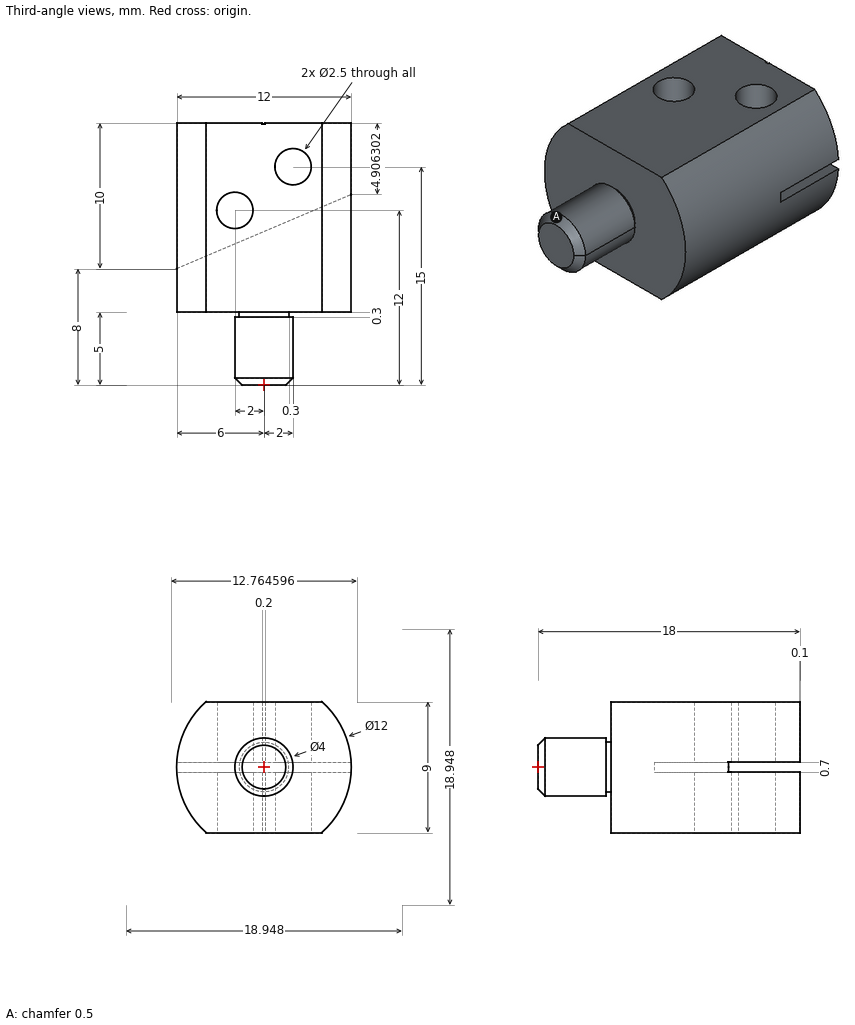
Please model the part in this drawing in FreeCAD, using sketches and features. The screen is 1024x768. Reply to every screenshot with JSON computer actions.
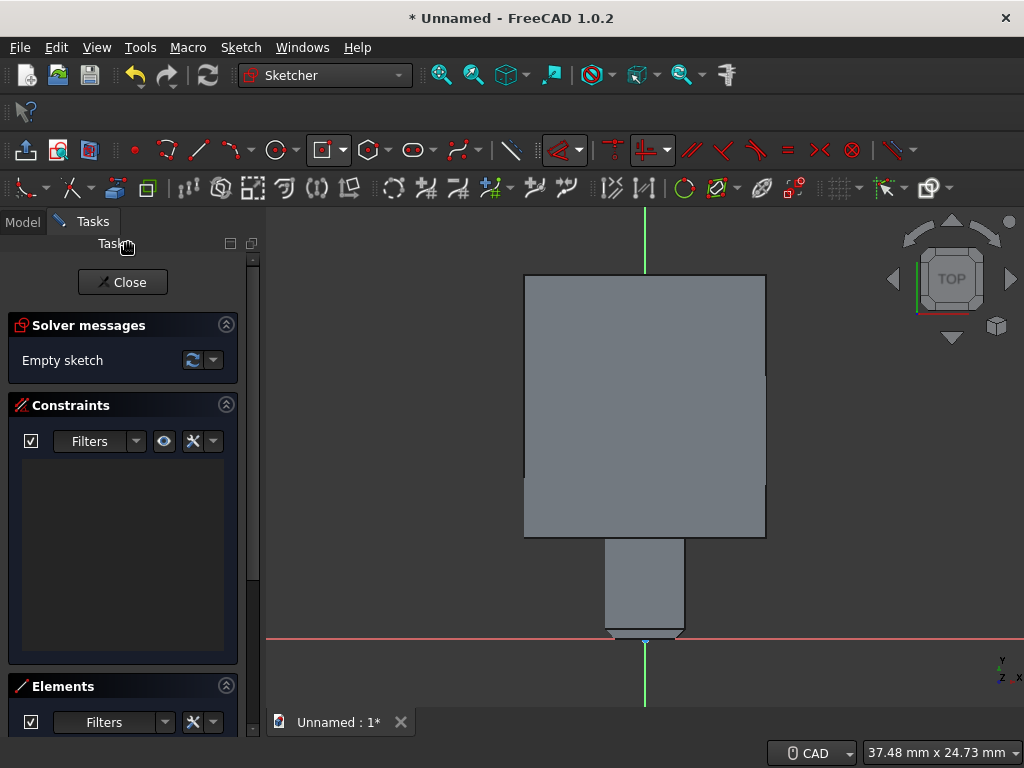
{"action": "left_click", "coordinate": [90, 150]}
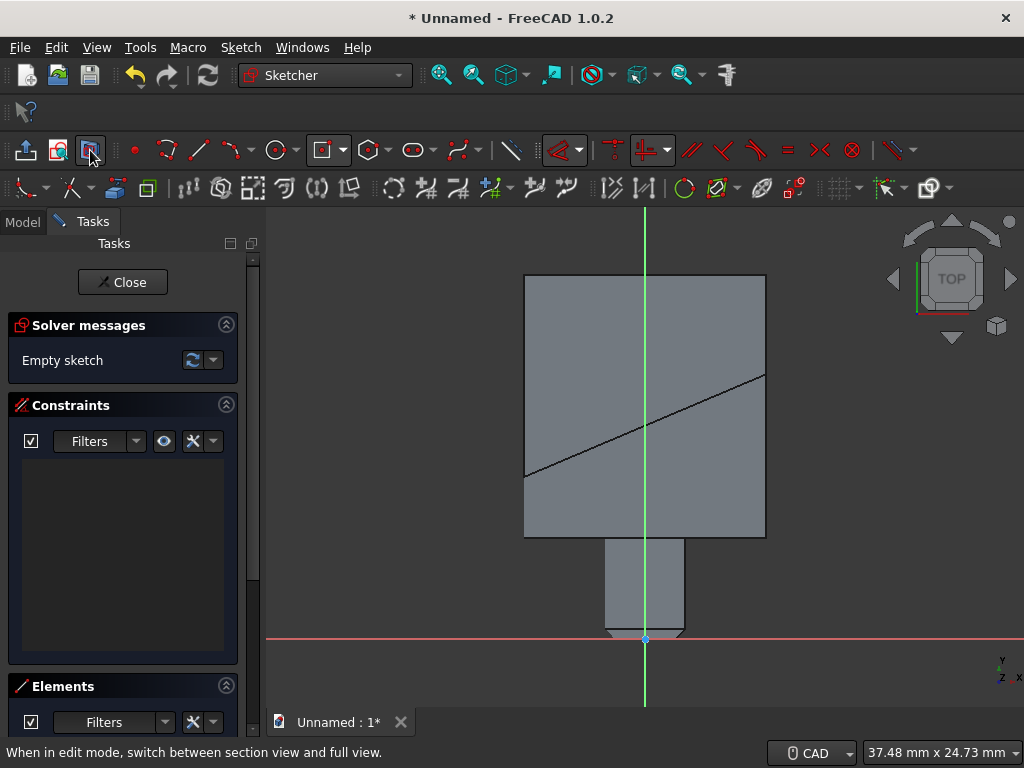
{"action": "scroll", "coordinate": [688, 545], "scroll_direction": "up", "scroll_amount": 15}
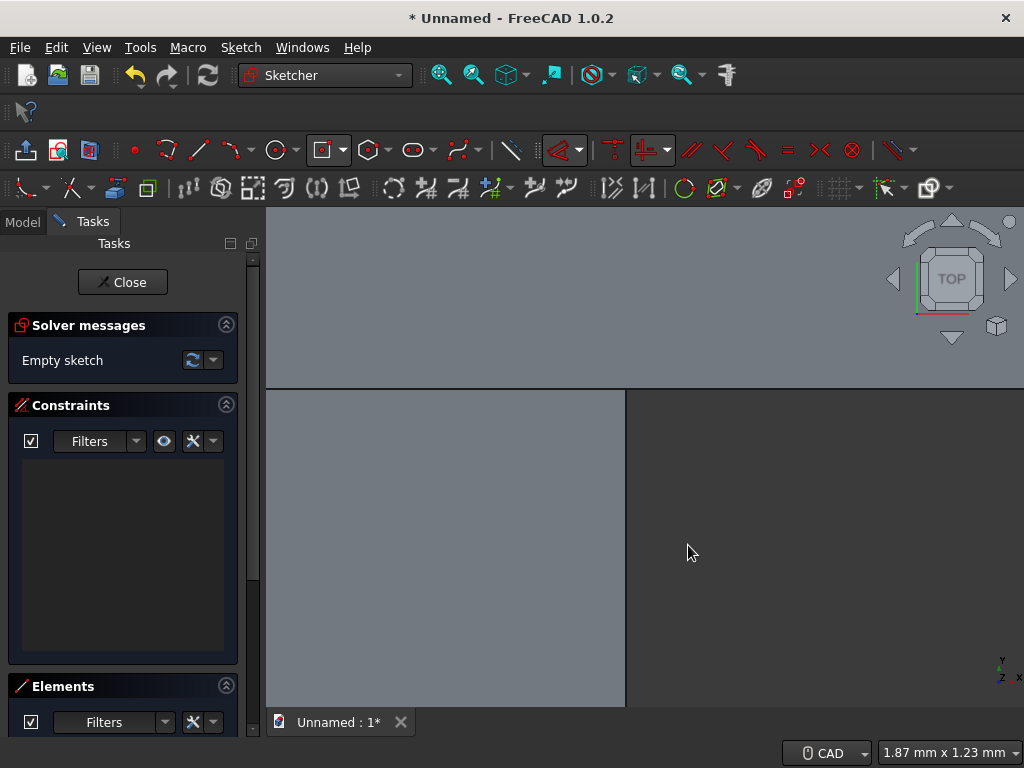
{"action": "scroll", "coordinate": [558, 446], "scroll_direction": "up", "scroll_amount": 5}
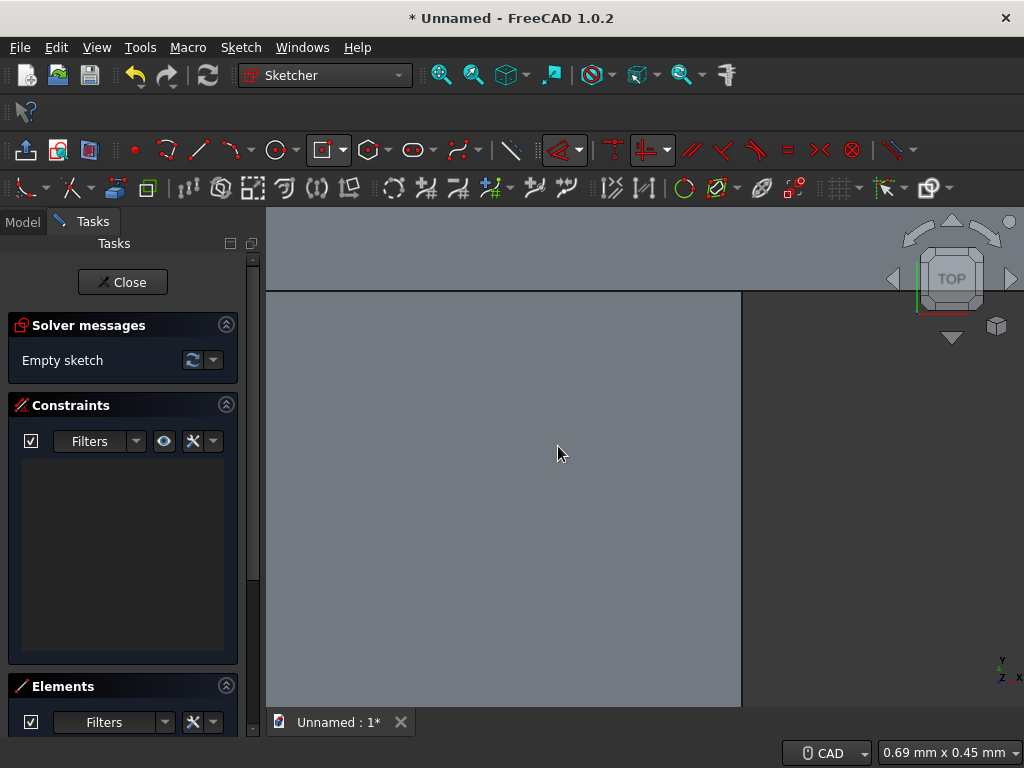
{"action": "left_click", "coordinate": [346, 150]}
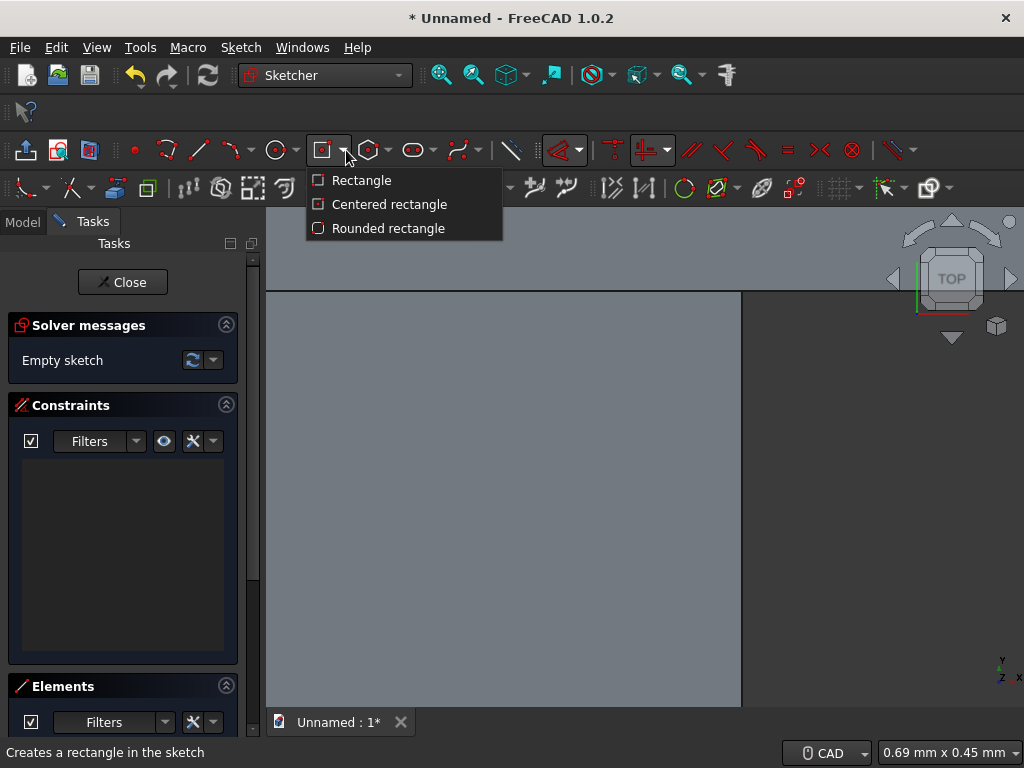
{"action": "left_click", "coordinate": [404, 180]}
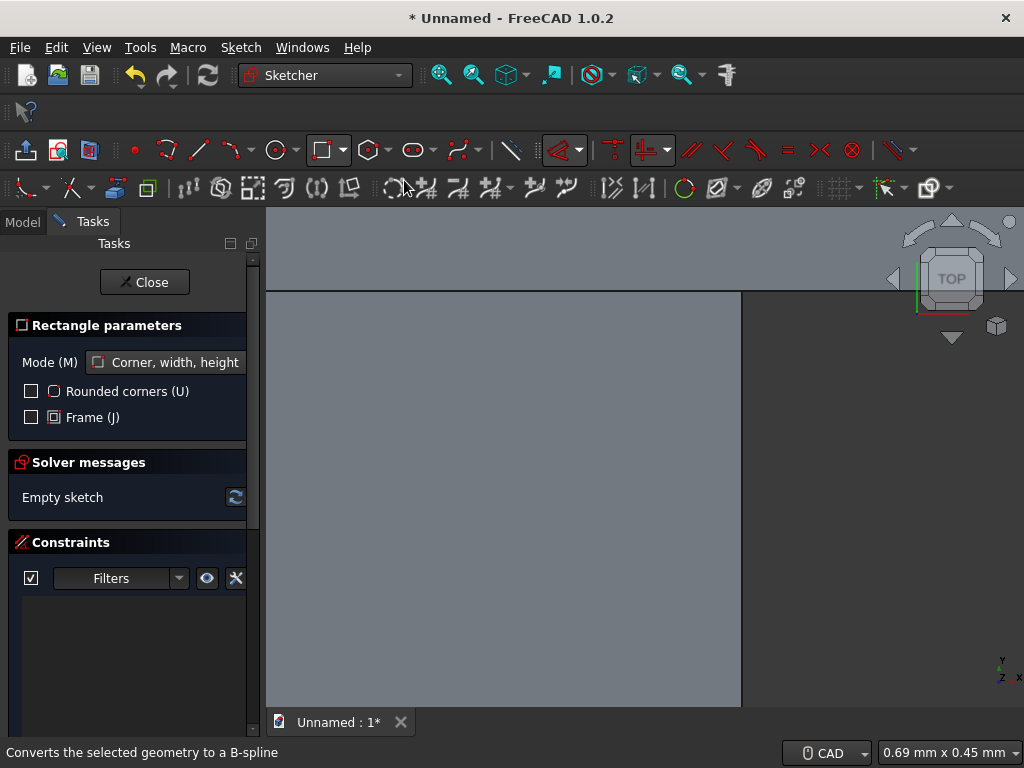
{"action": "left_click", "coordinate": [411, 291]}
{"action": "left_click", "coordinate": [742, 622]}
{"action": "key", "text": "Escape"}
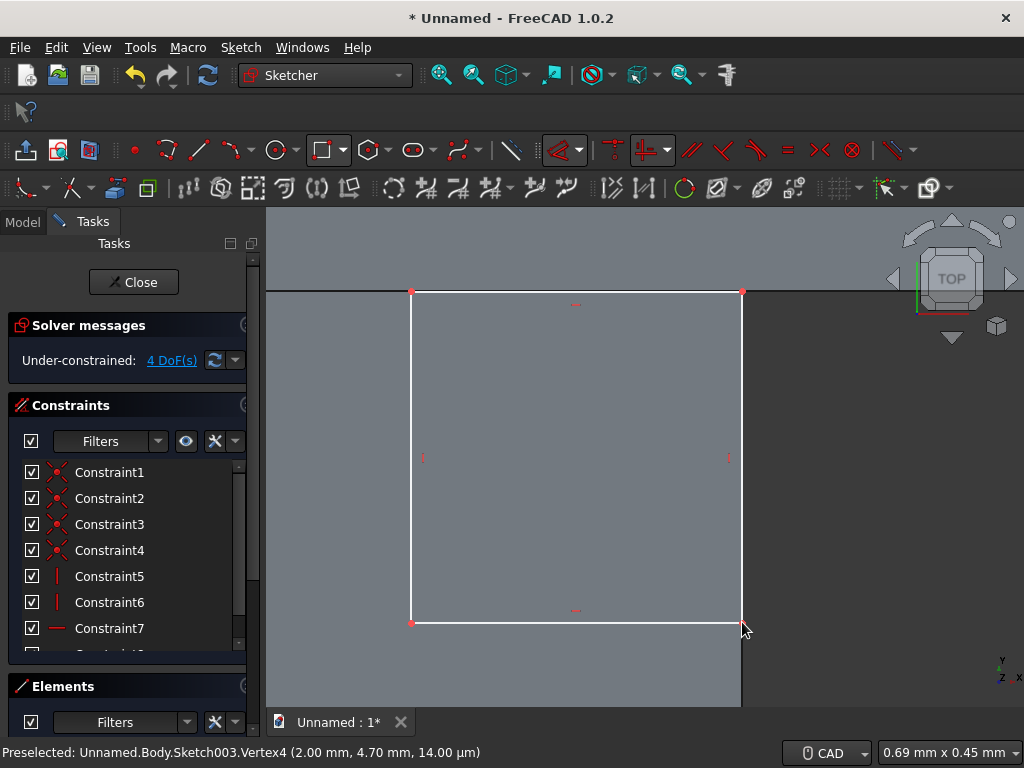
{"action": "left_click", "coordinate": [411, 292]}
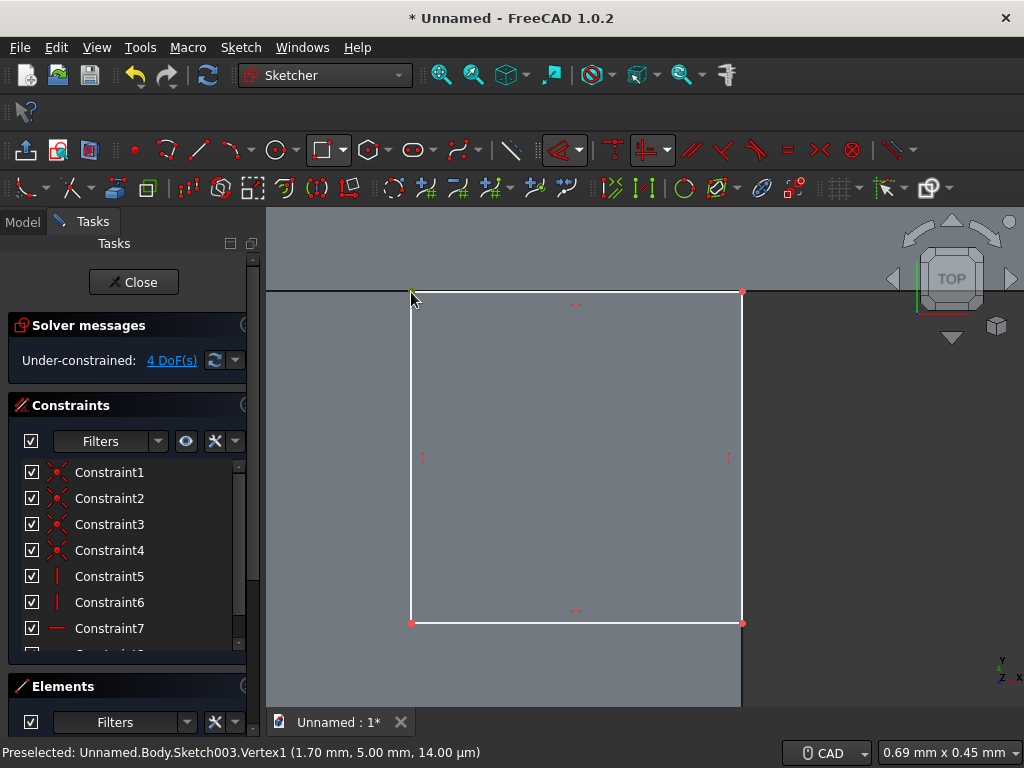
{"action": "key", "text": "i"}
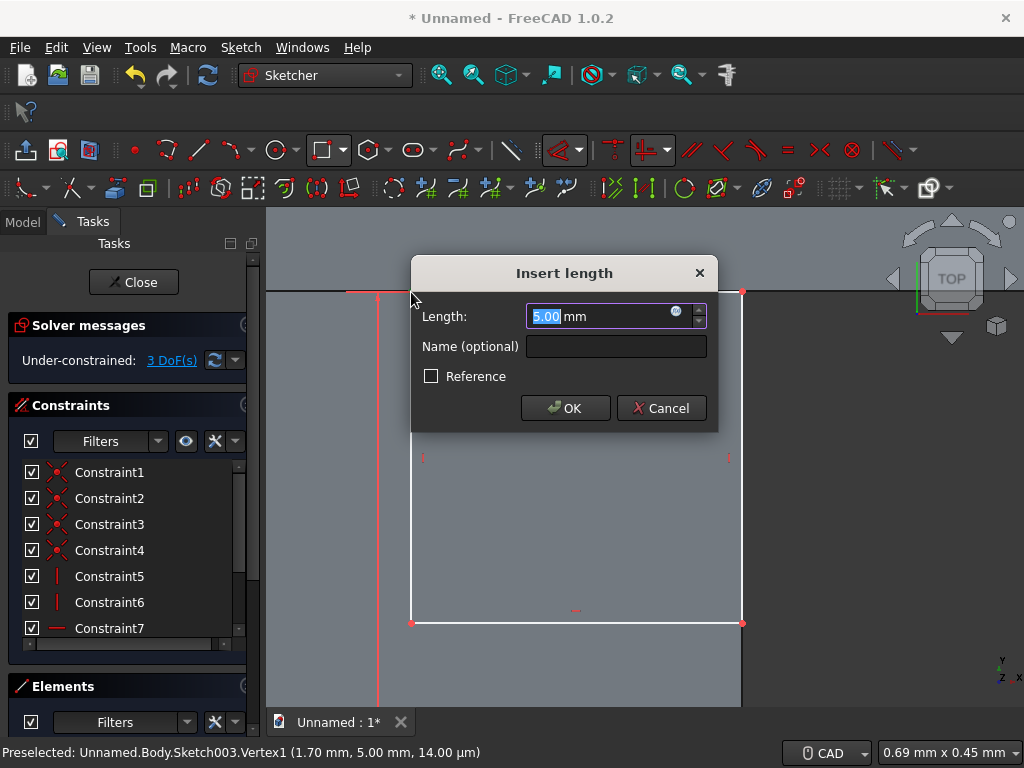
{"action": "type", "text": "5"}
{"action": "key", "text": "Return"}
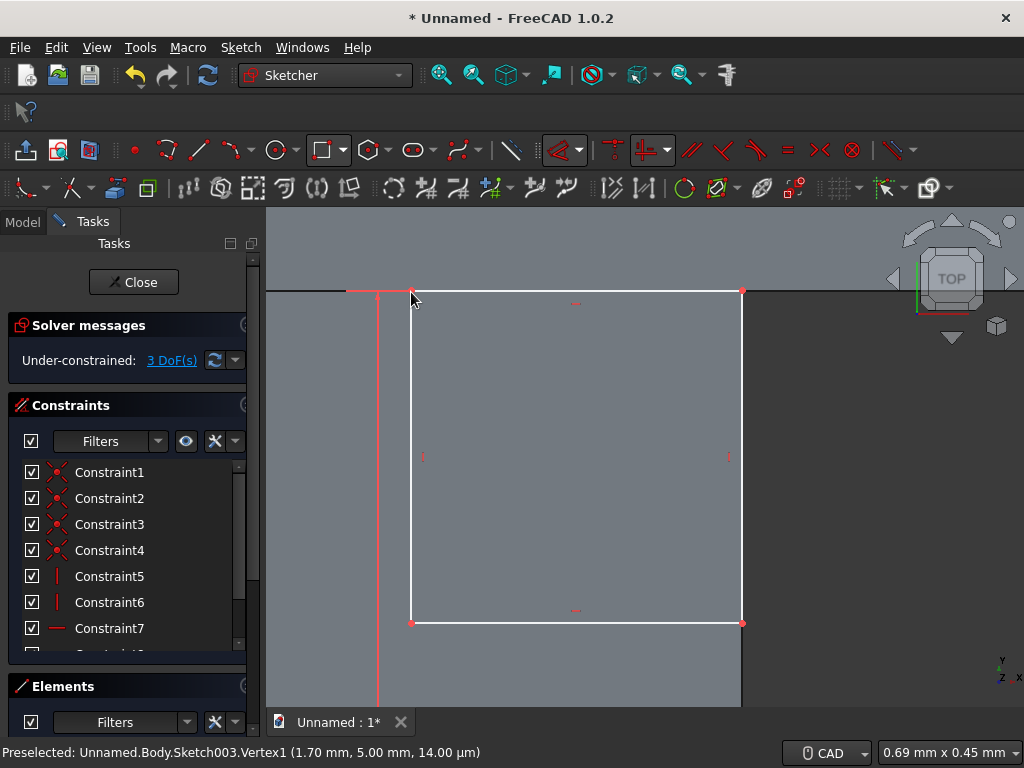
{"action": "left_click", "coordinate": [742, 623]}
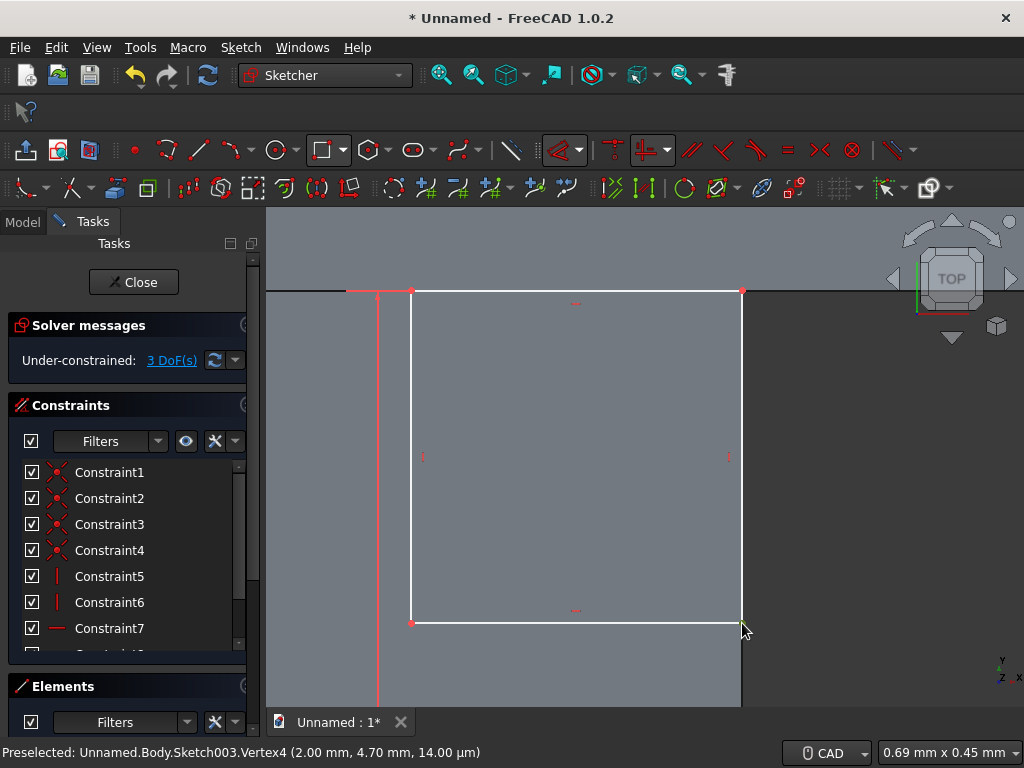
{"action": "left_click", "coordinate": [582, 150]}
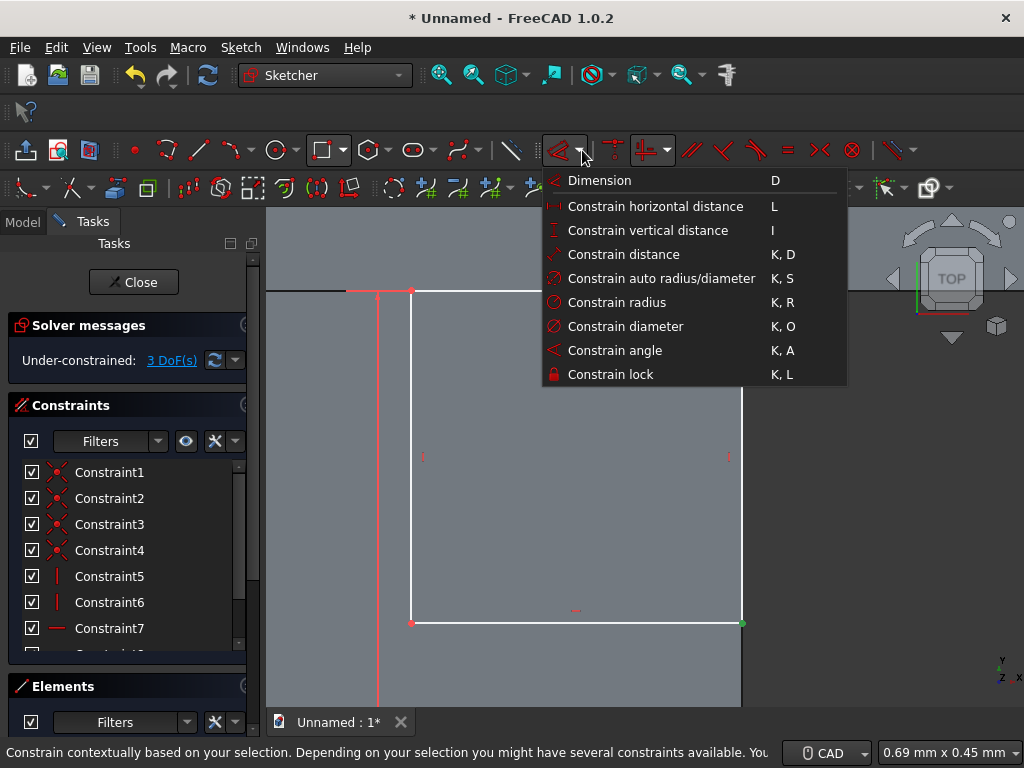
{"action": "left_click", "coordinate": [695, 206]}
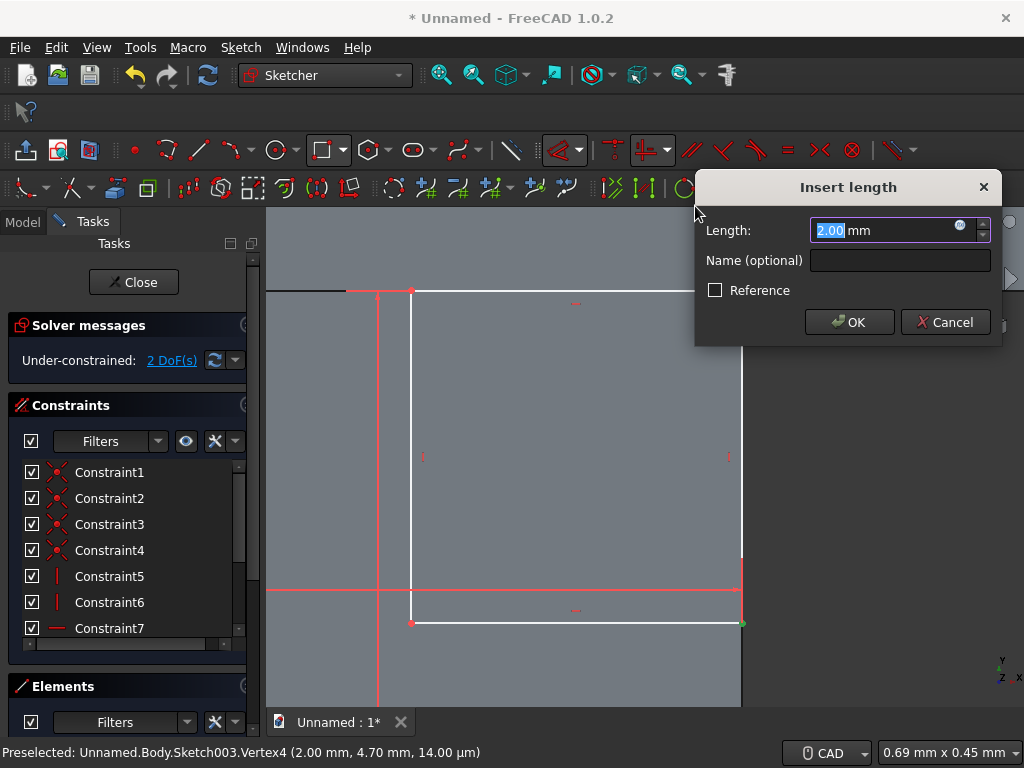
{"action": "type", "text": "2"}
{"action": "key", "text": "Return"}